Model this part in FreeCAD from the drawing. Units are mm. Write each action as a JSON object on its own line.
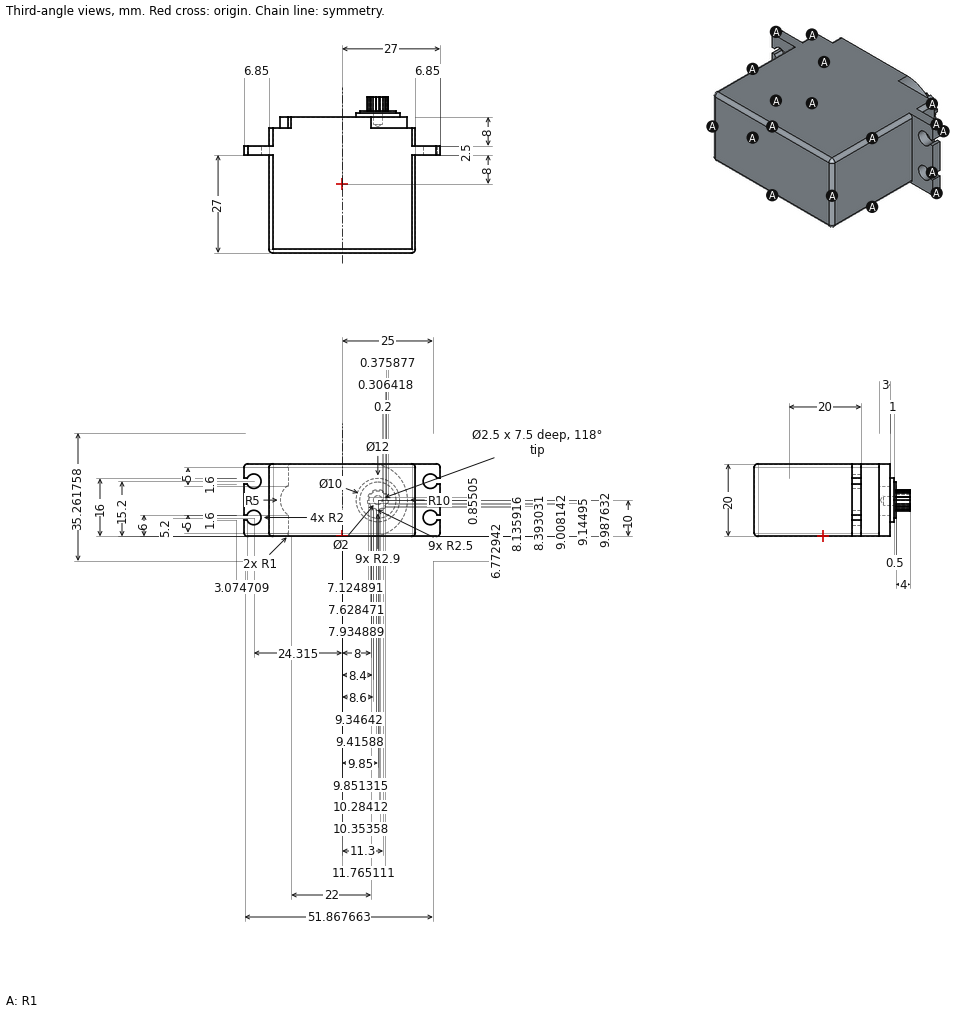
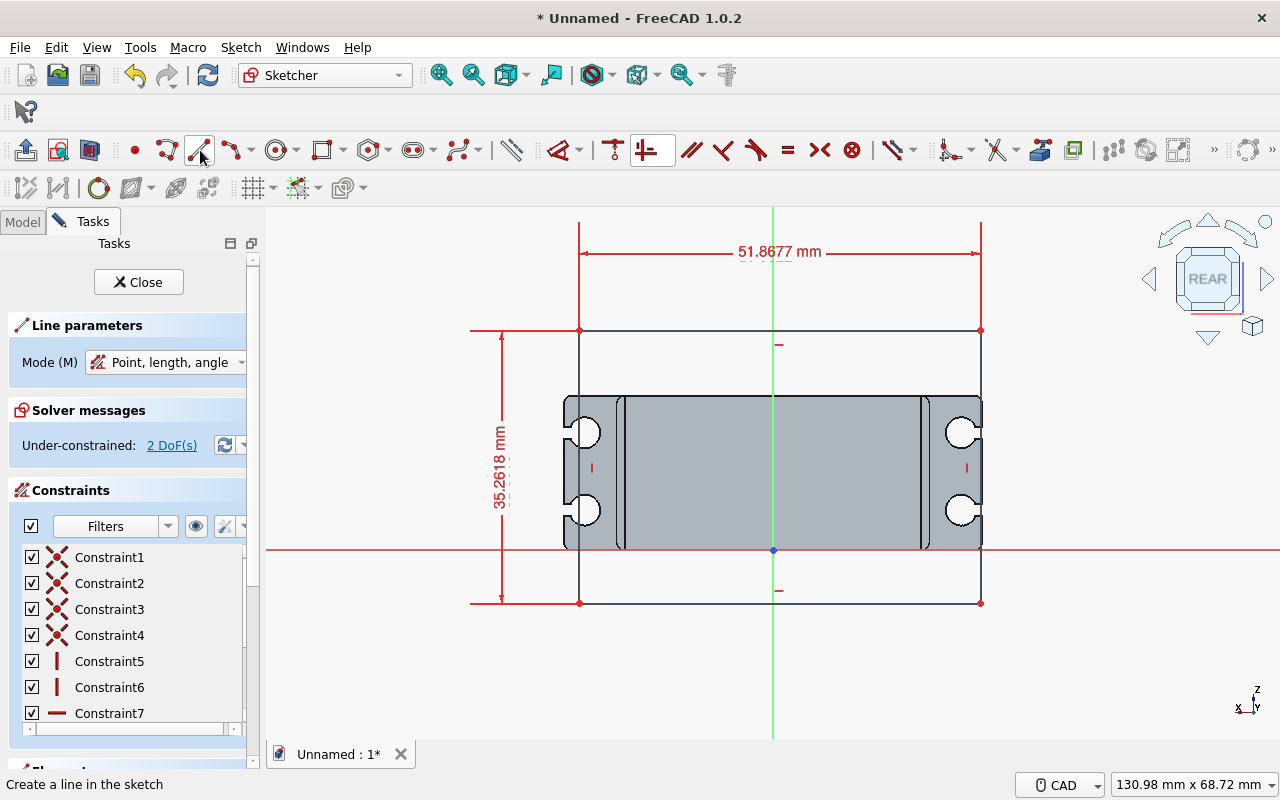
{"action": "left_click", "coordinate": [881, 550]}
{"action": "left_click", "coordinate": [711, 541]}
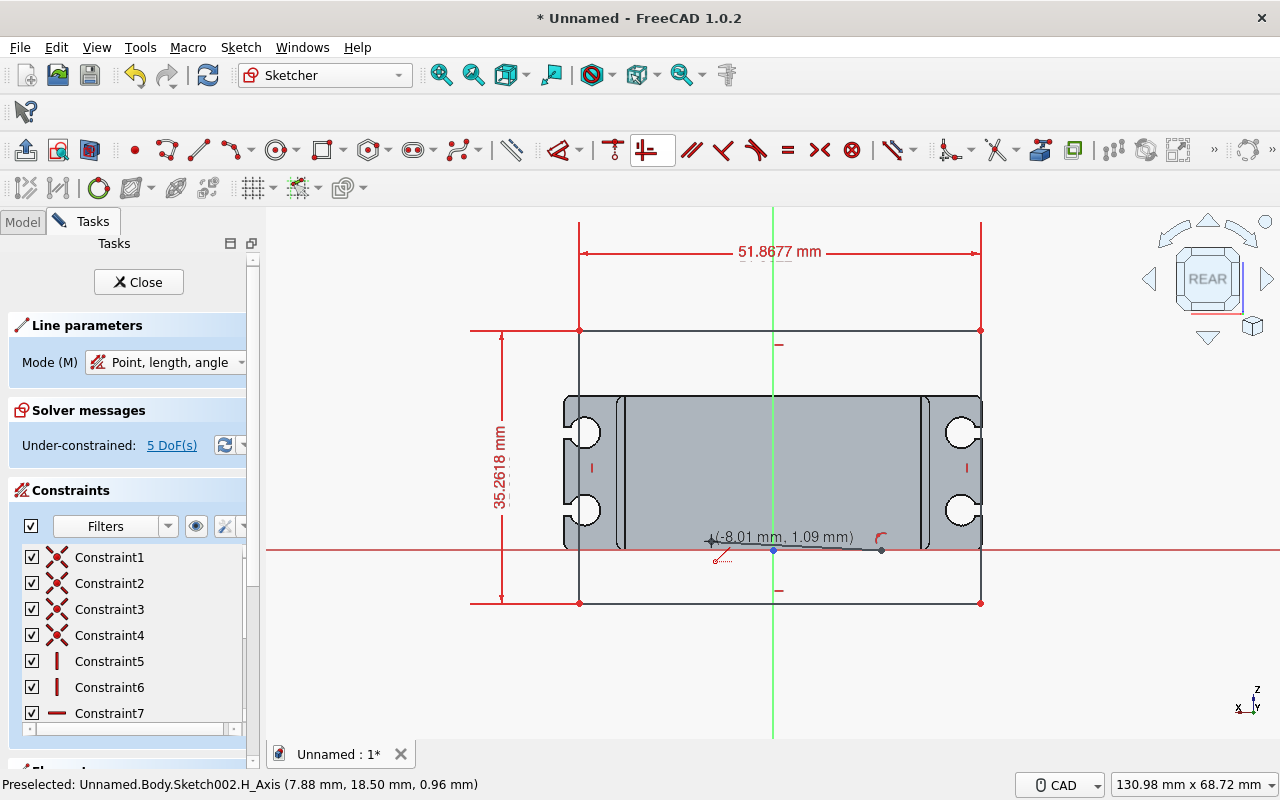
{"action": "left_click", "coordinate": [711, 396]}
{"action": "left_click", "coordinate": [881, 396]}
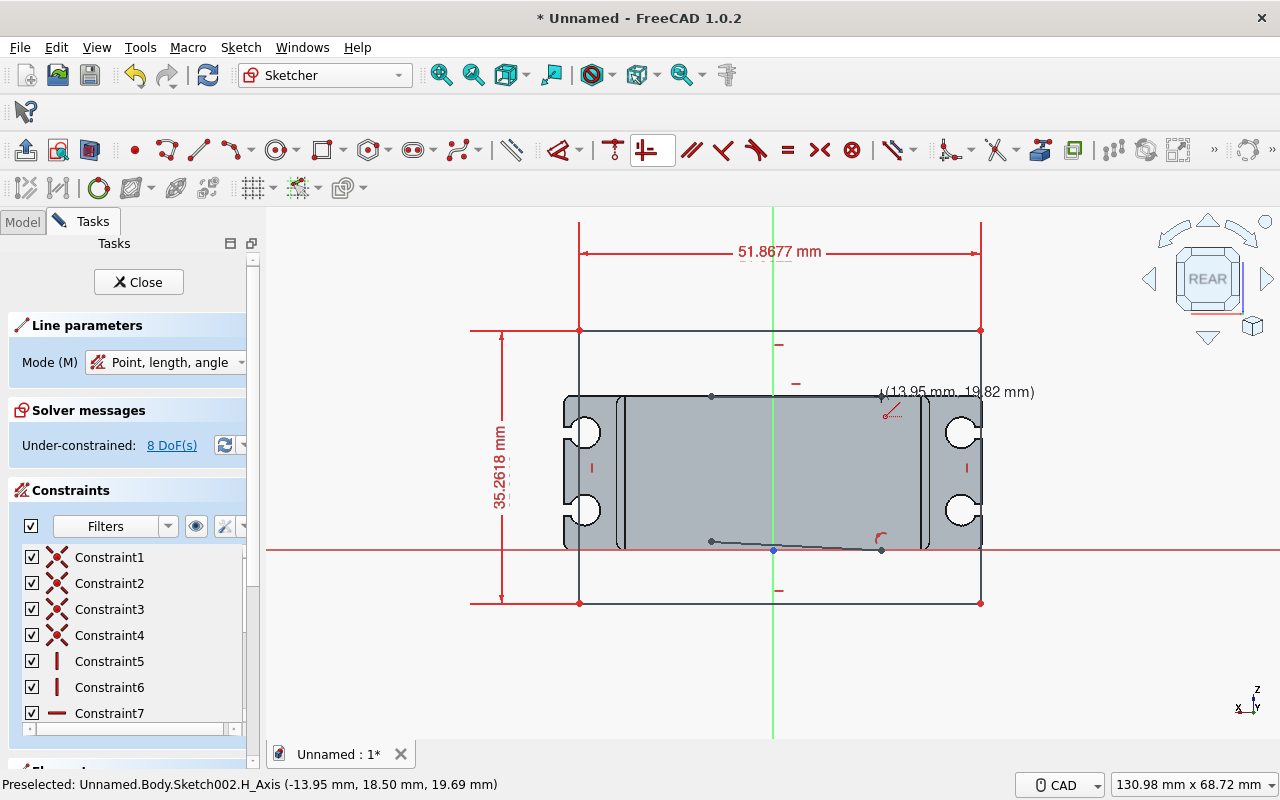
{"action": "scroll", "coordinate": [889, 403], "scroll_direction": "up", "scroll_amount": 2}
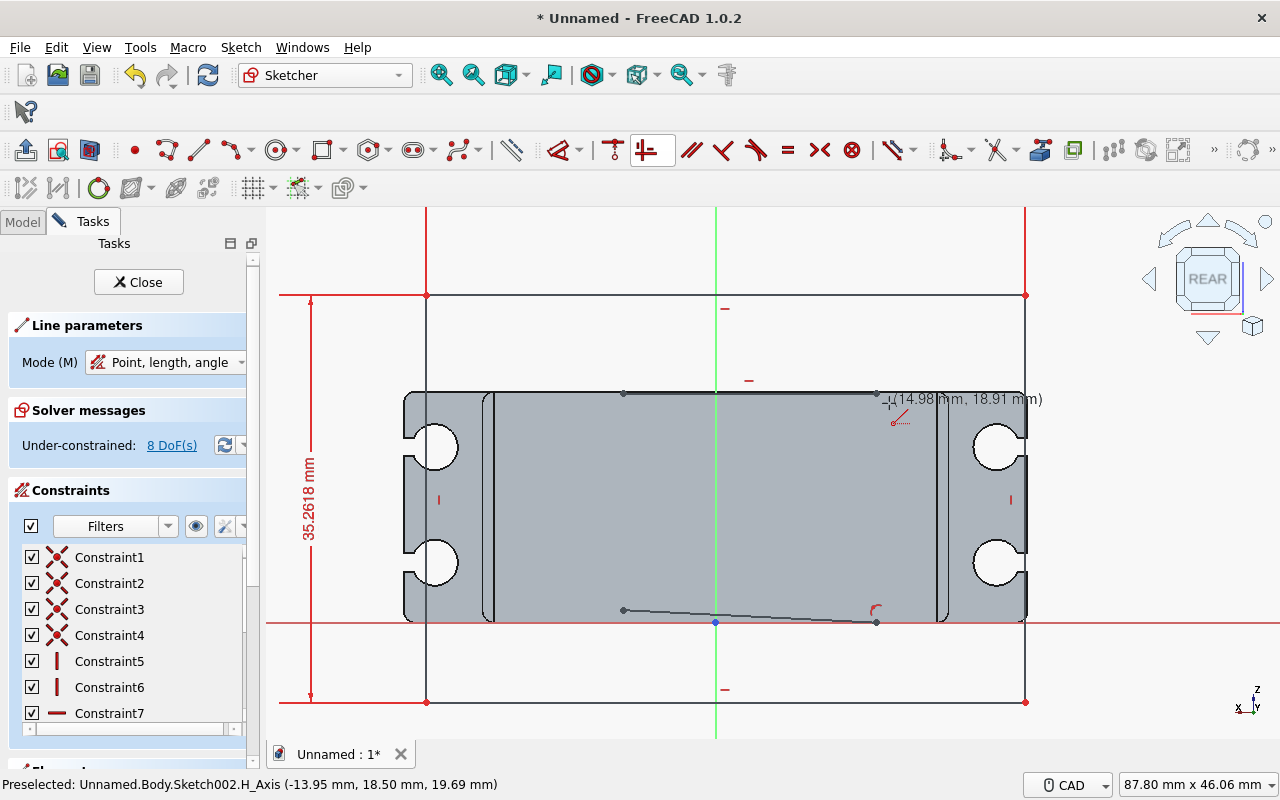
{"action": "left_click", "coordinate": [889, 403]}
{"action": "left_click", "coordinate": [889, 461]}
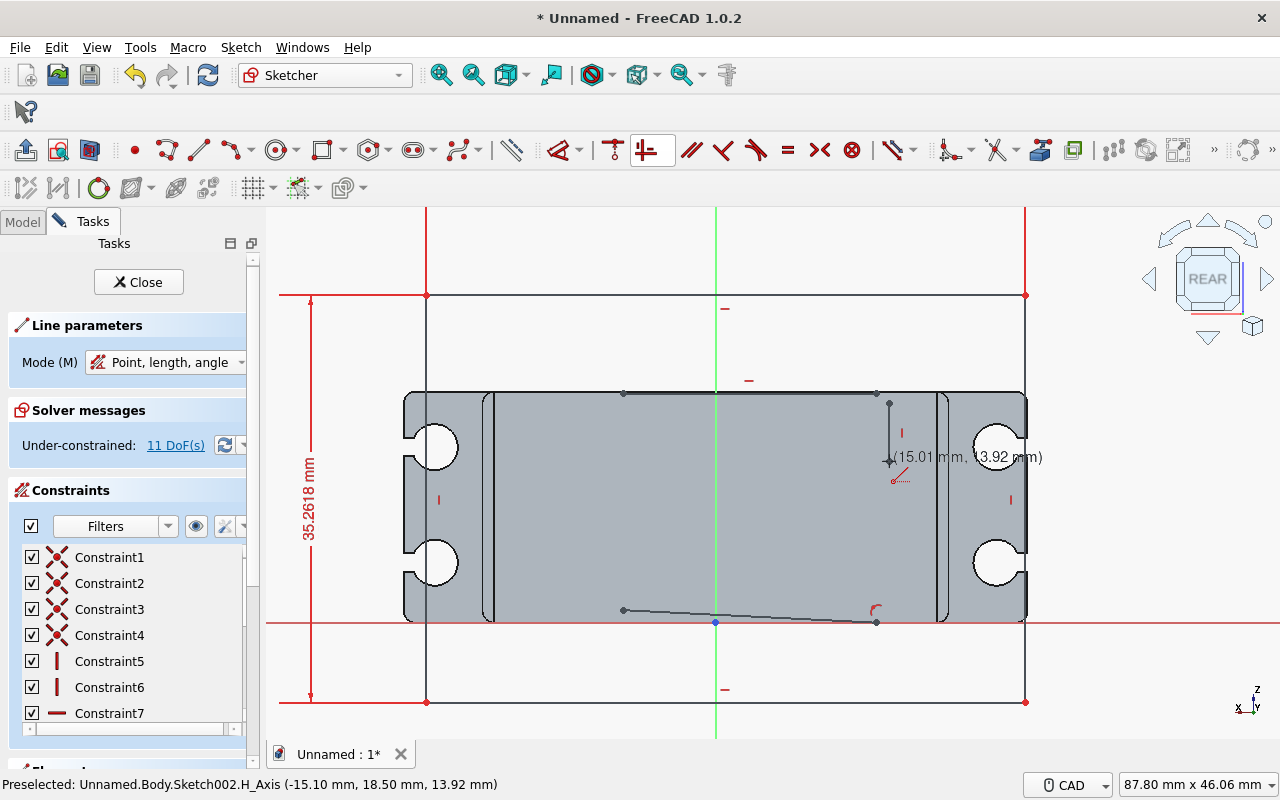
{"action": "left_click", "coordinate": [889, 553]}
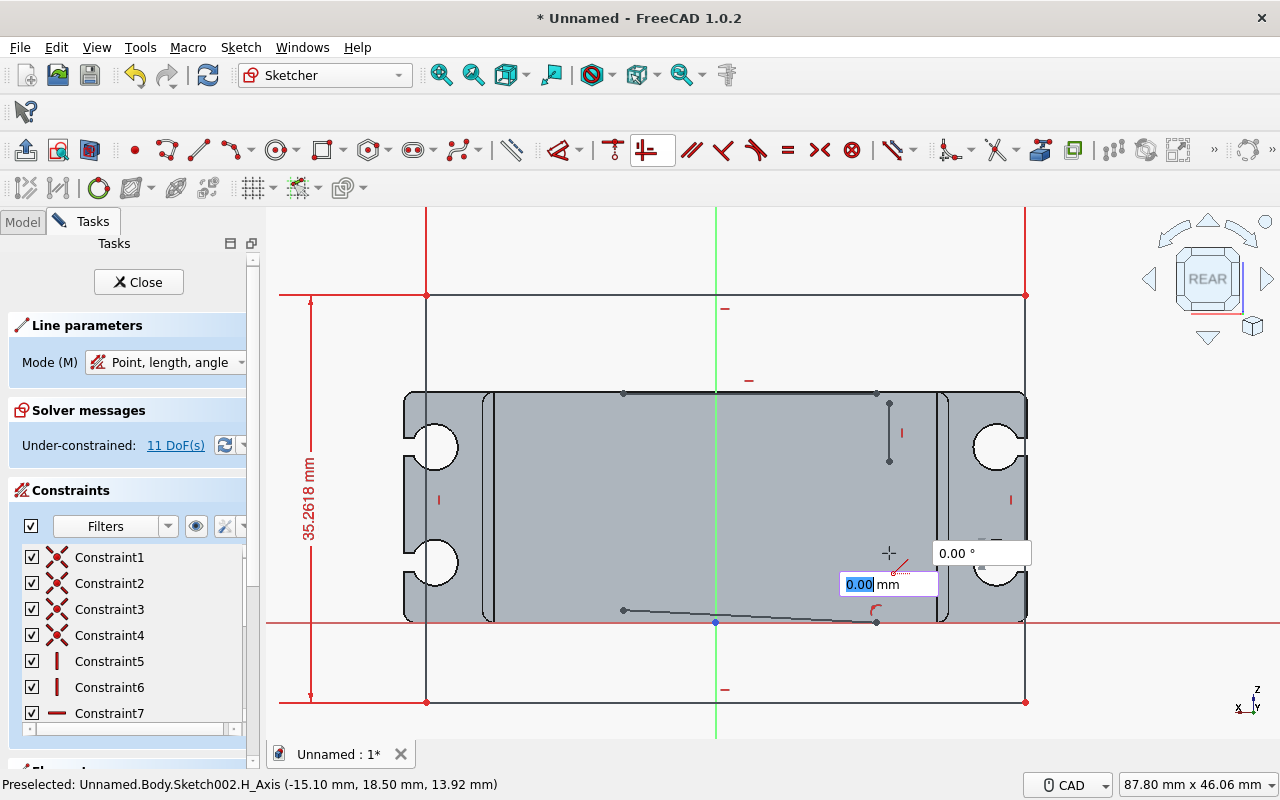
{"action": "scroll", "coordinate": [889, 611], "scroll_direction": "up", "scroll_amount": 2}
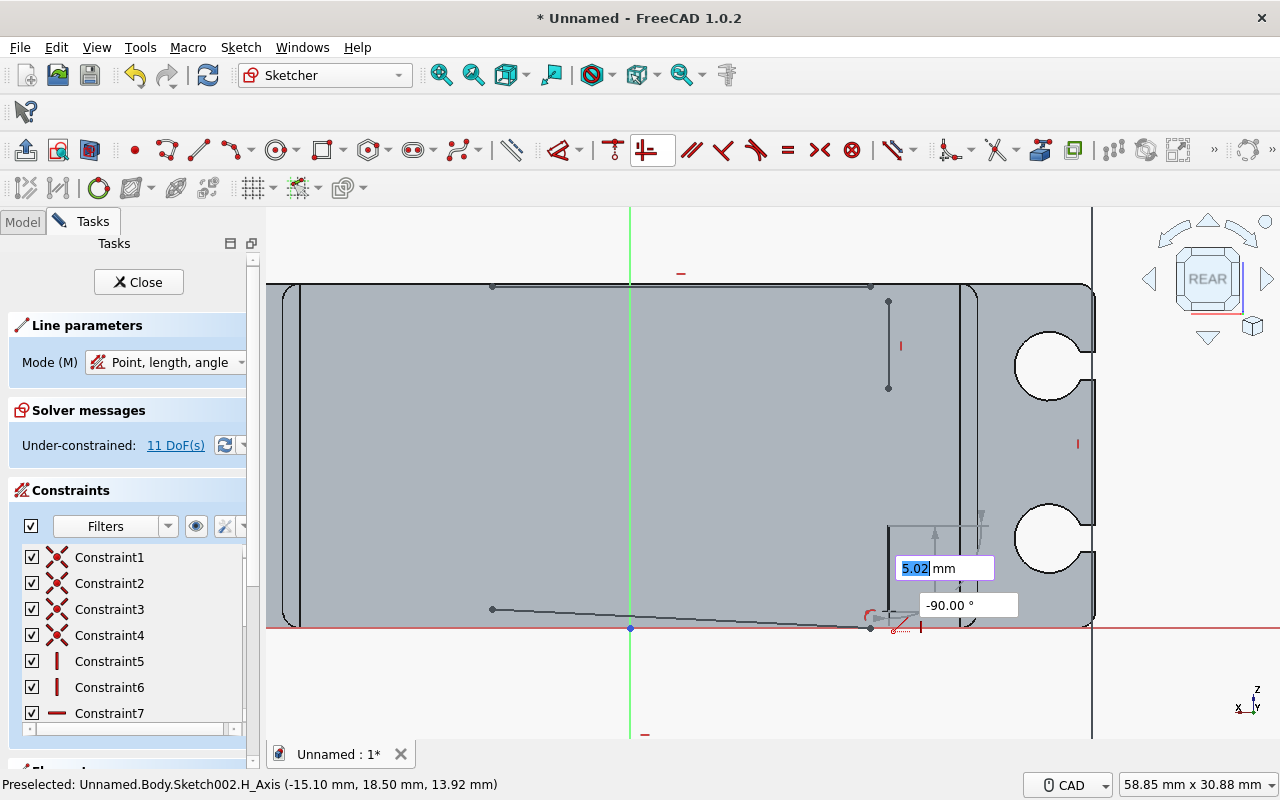
{"action": "left_click", "coordinate": [889, 611]}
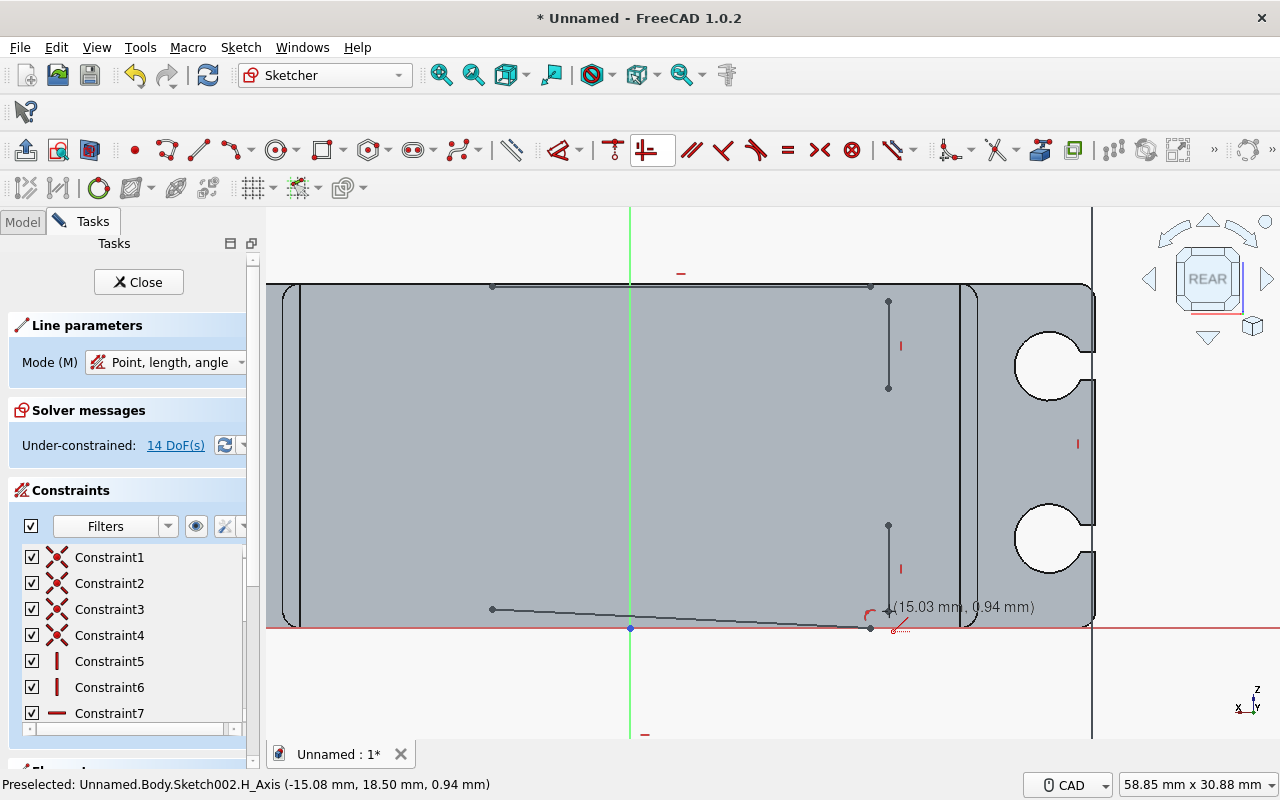
{"action": "left_click", "coordinate": [232, 150]}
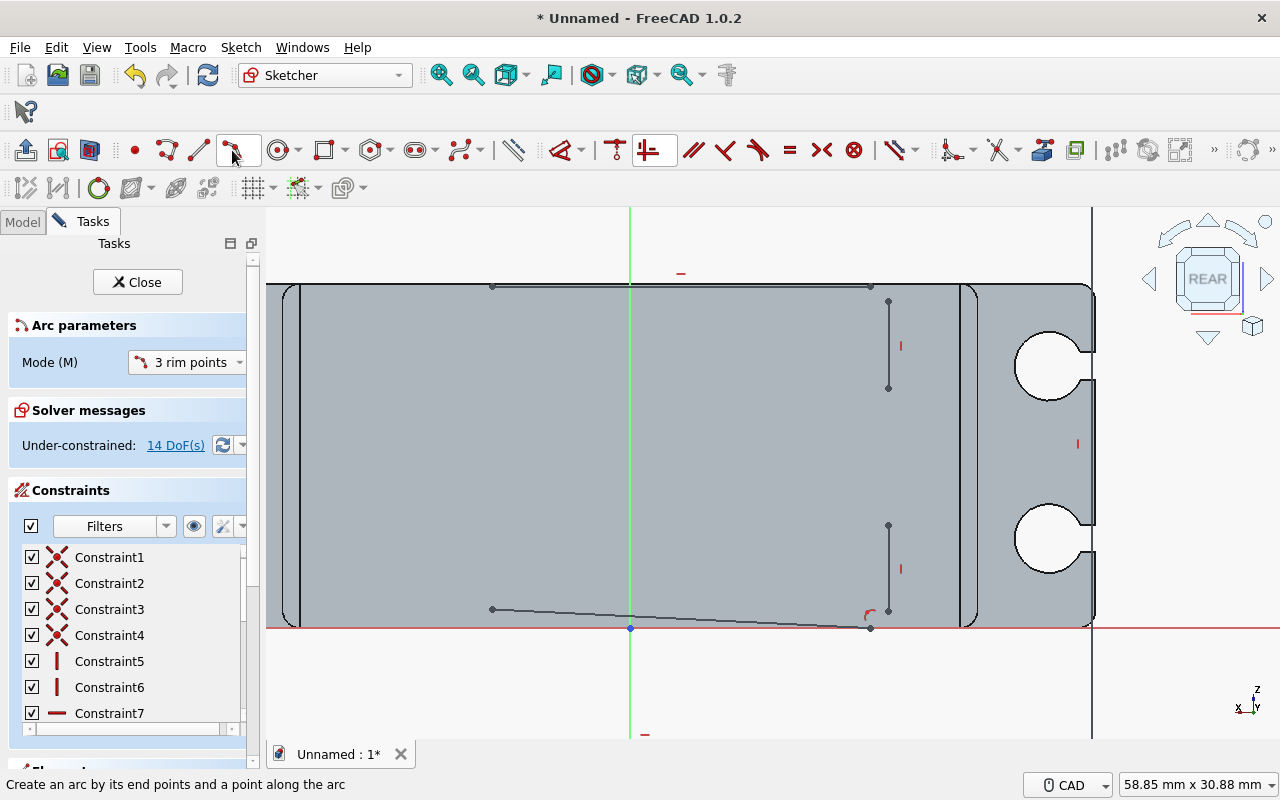
{"action": "left_click", "coordinate": [492, 609]}
{"action": "left_click", "coordinate": [492, 287]}
{"action": "left_click", "coordinate": [320, 456]}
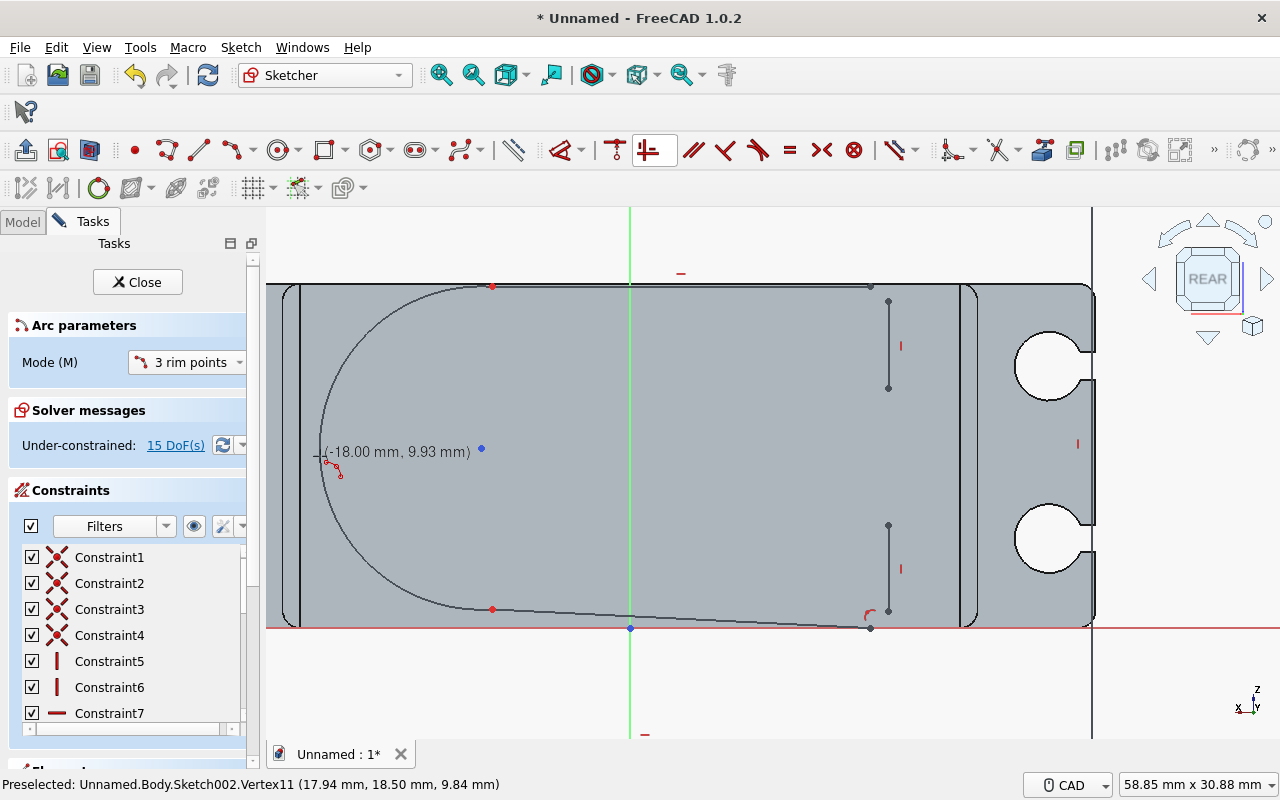
{"action": "left_click", "coordinate": [870, 287]}
{"action": "left_click", "coordinate": [889, 302]}